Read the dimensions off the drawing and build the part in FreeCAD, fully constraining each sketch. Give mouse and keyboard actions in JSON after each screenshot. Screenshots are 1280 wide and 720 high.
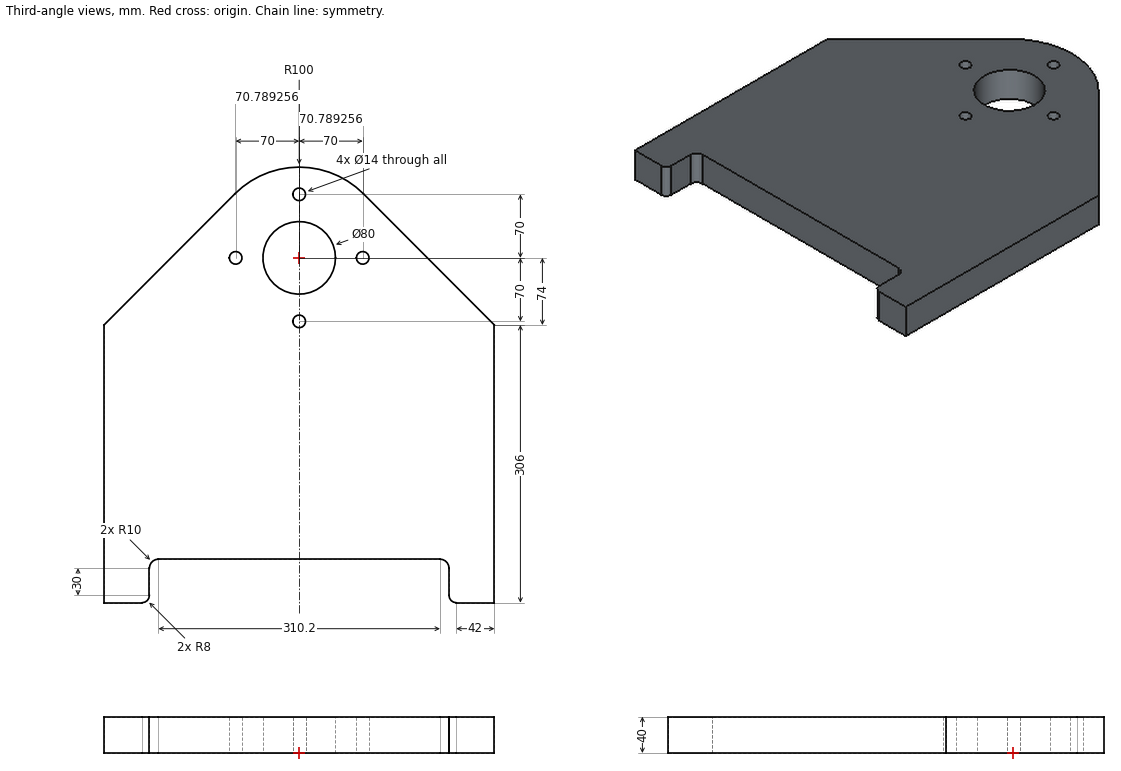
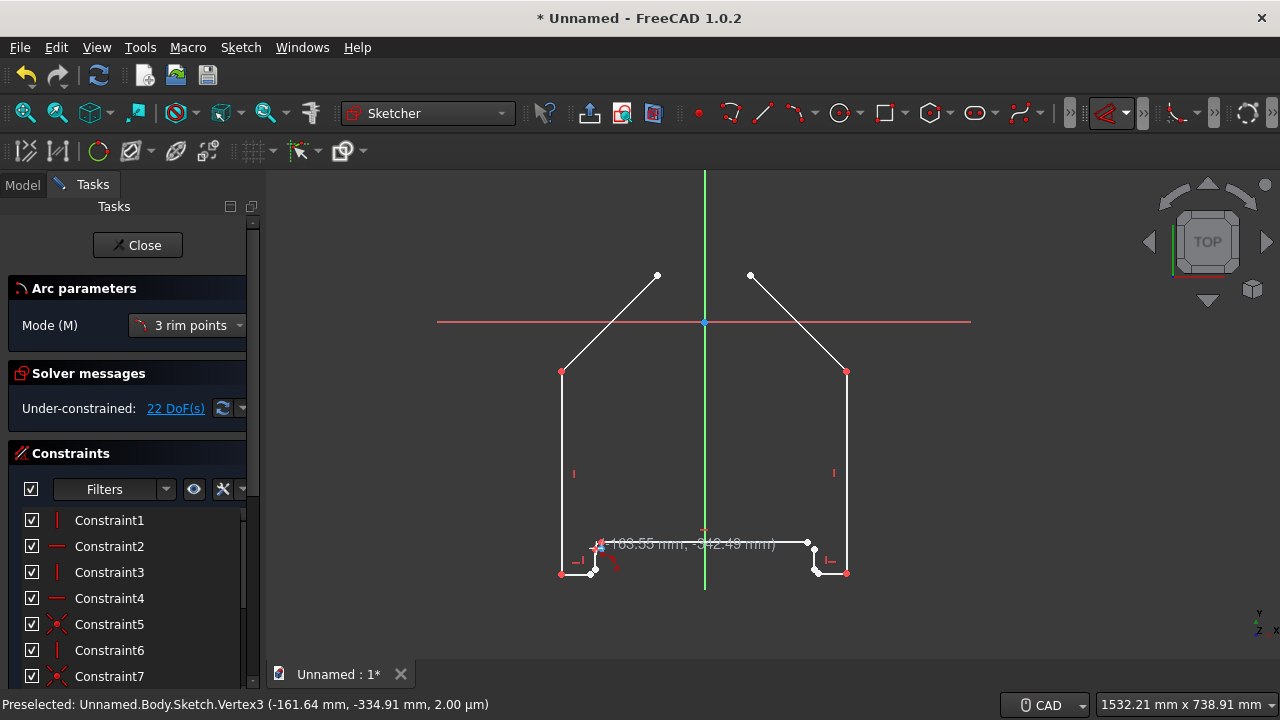
{"action": "scroll", "coordinate": [807, 542], "scroll_direction": "up", "scroll_amount": 3}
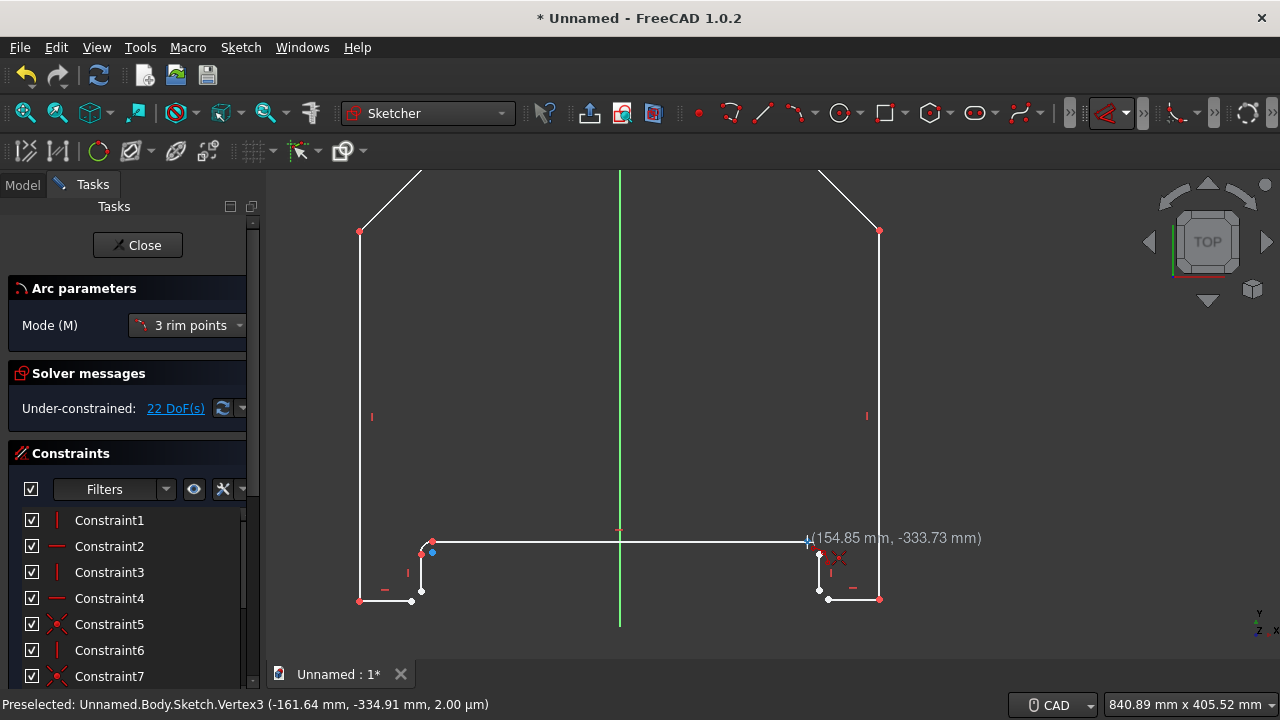
{"action": "left_click", "coordinate": [807, 542]}
{"action": "left_click", "coordinate": [819, 555]}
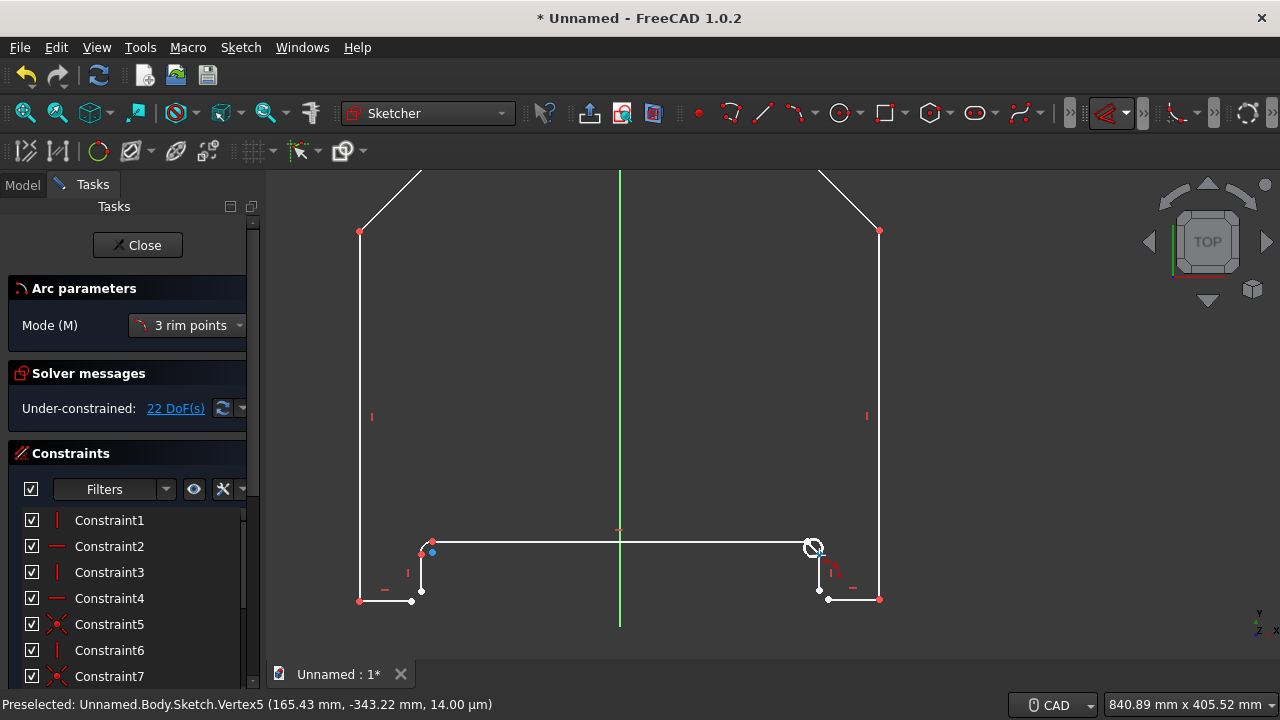
{"action": "scroll", "coordinate": [815, 545], "scroll_direction": "up", "scroll_amount": 8}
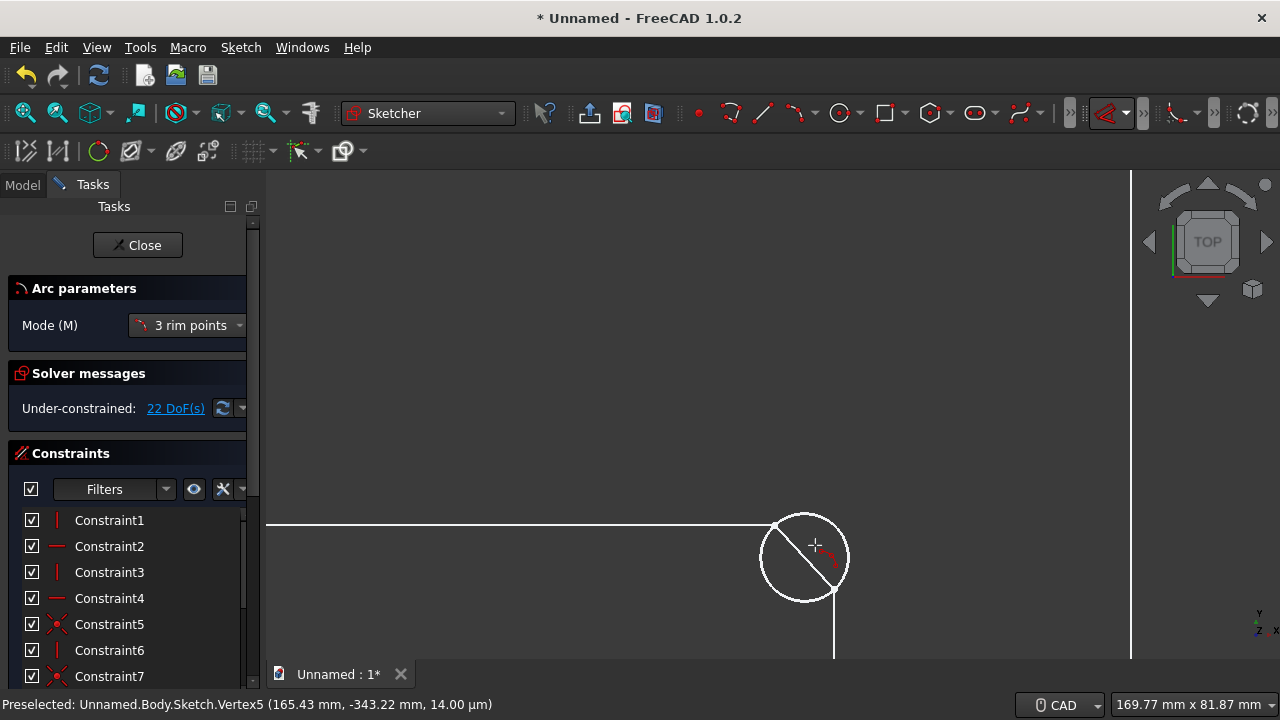
{"action": "left_click", "coordinate": [815, 540]}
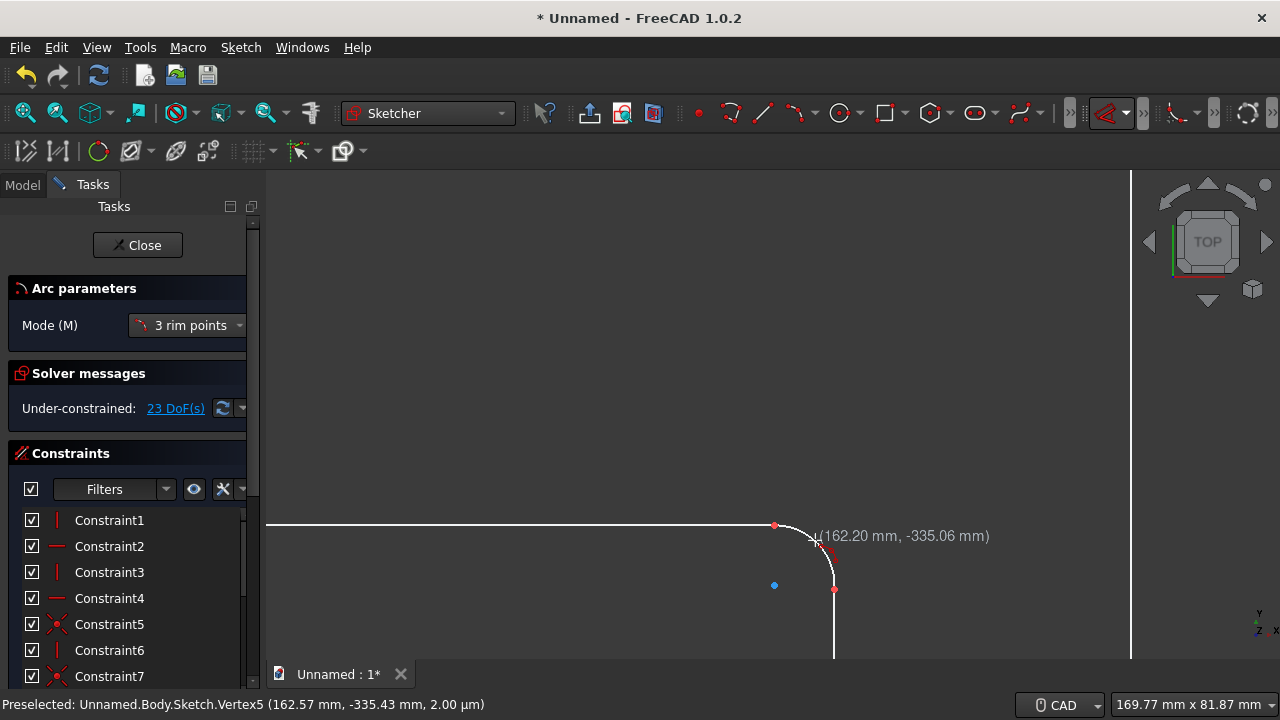
{"action": "scroll", "coordinate": [811, 544], "scroll_direction": "down", "scroll_amount": 11}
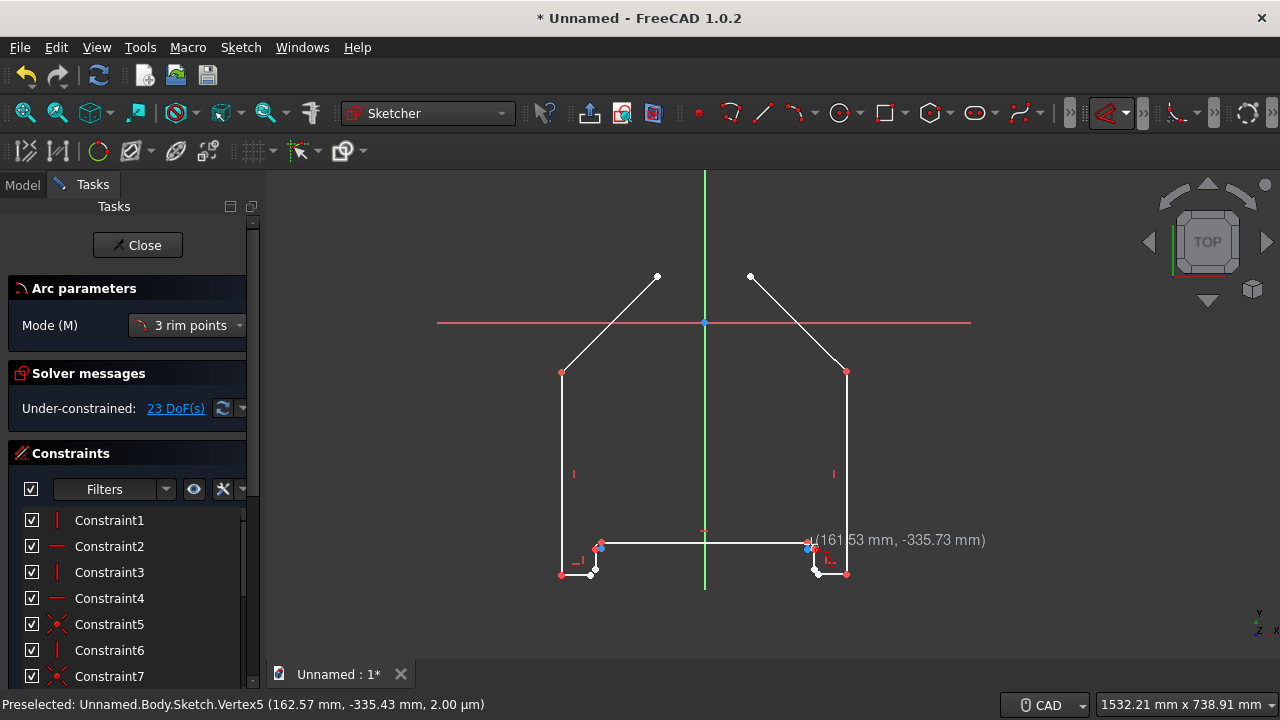
{"action": "scroll", "coordinate": [814, 569], "scroll_direction": "up", "scroll_amount": 4}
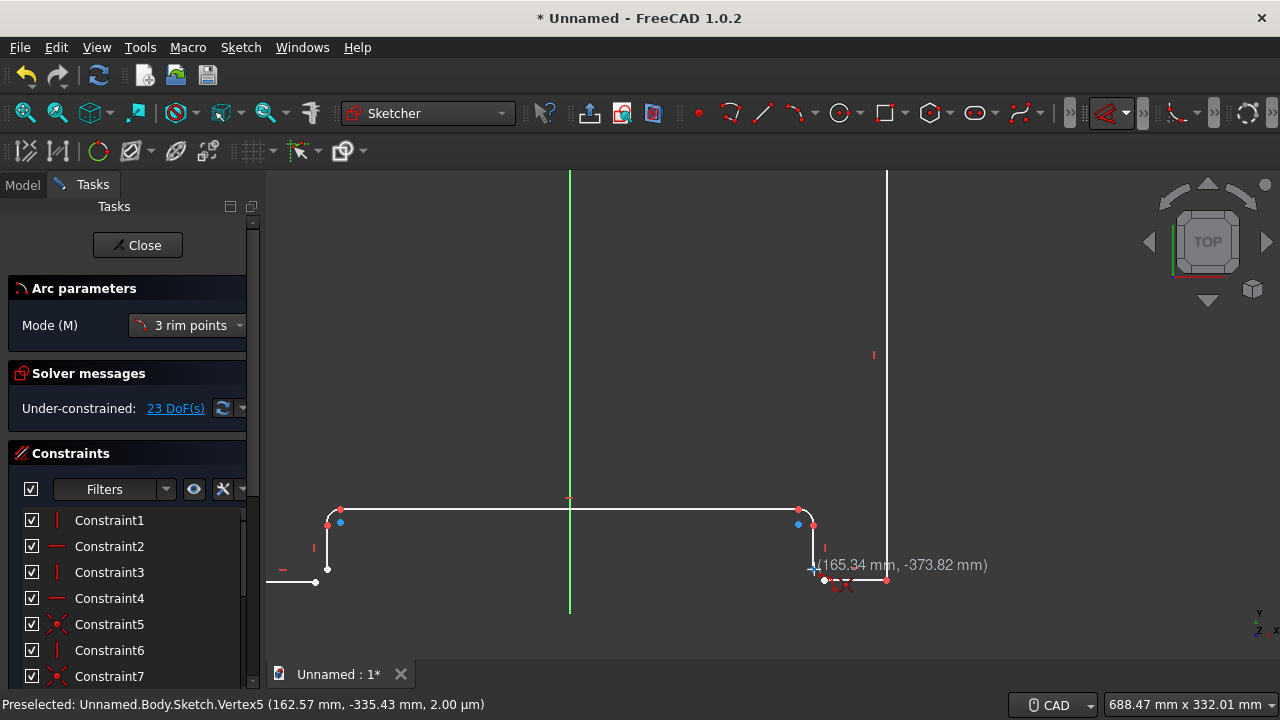
{"action": "left_click", "coordinate": [813, 569]}
{"action": "left_click", "coordinate": [824, 580]}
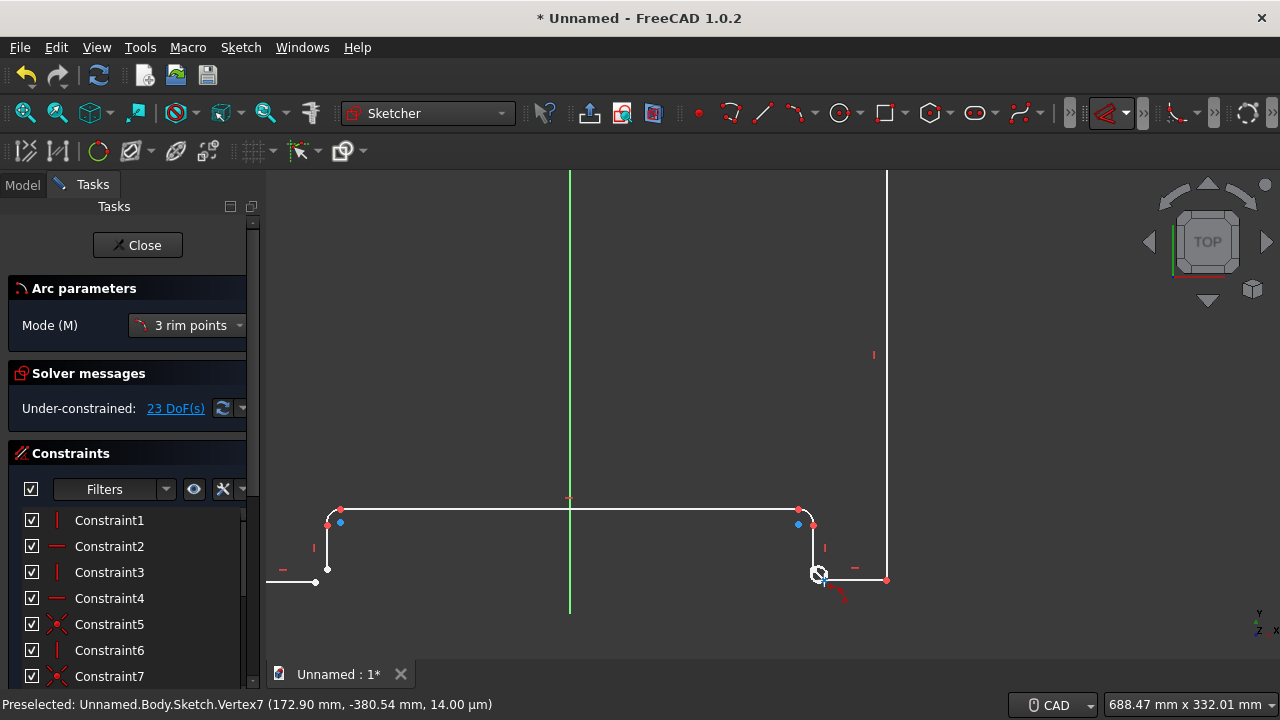
{"action": "scroll", "coordinate": [816, 576], "scroll_direction": "up", "scroll_amount": 8}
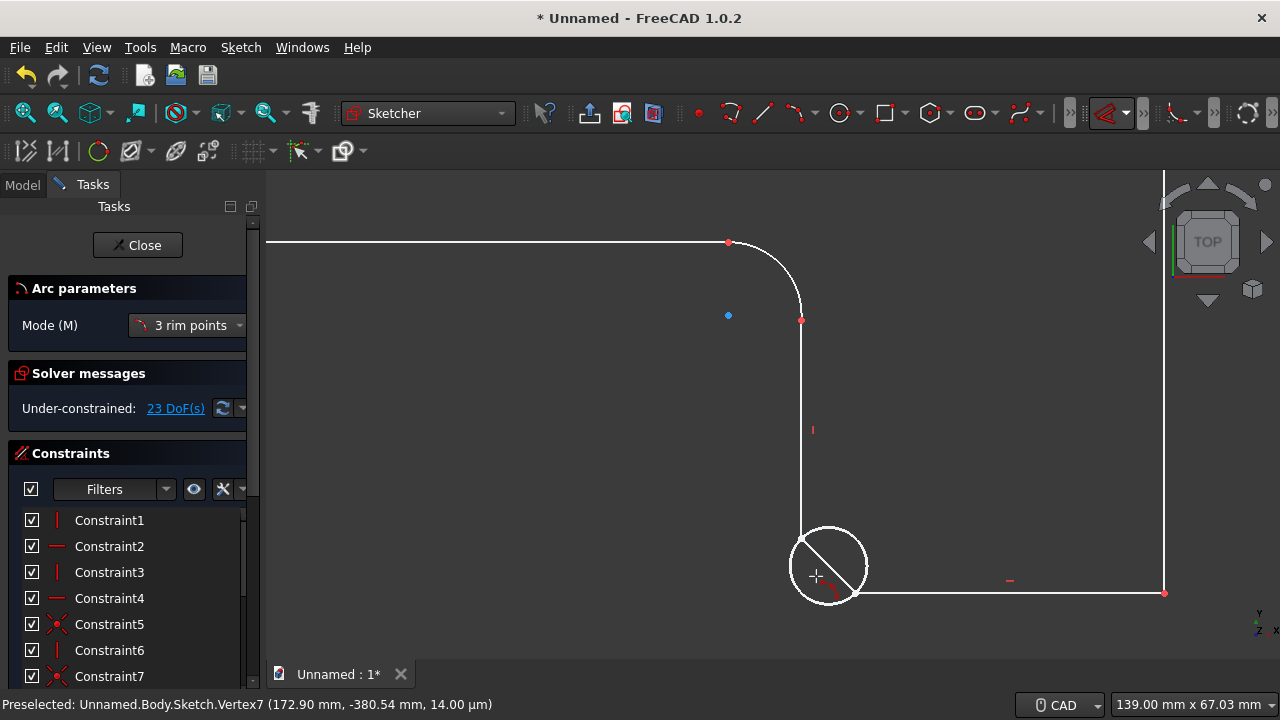
{"action": "left_click", "coordinate": [816, 572]}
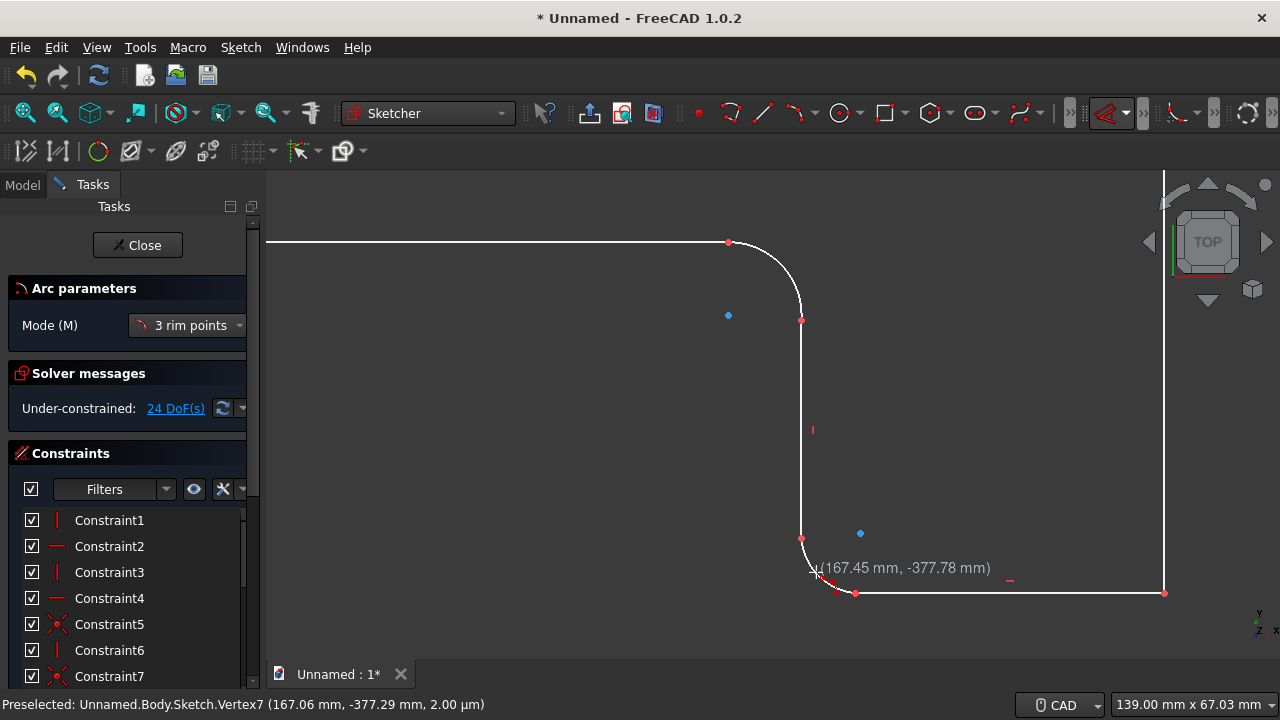
{"action": "scroll", "coordinate": [815, 572], "scroll_direction": "down", "scroll_amount": 12}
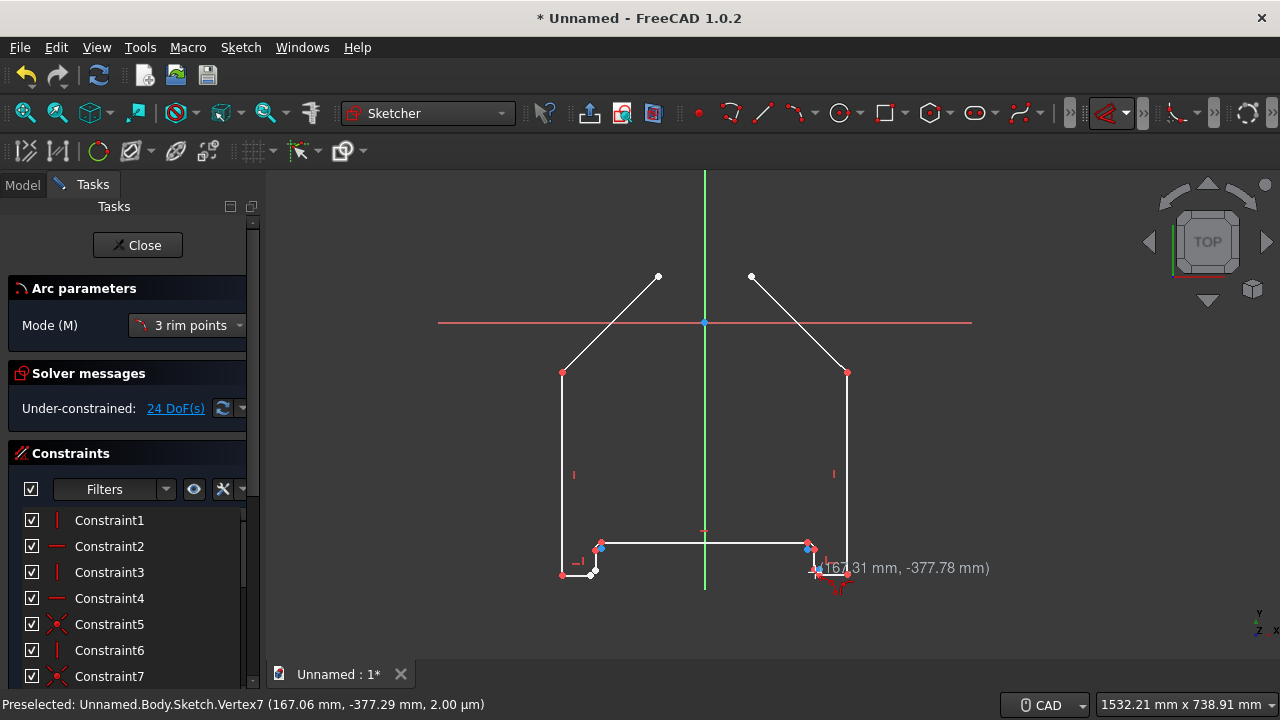
{"action": "left_click", "coordinate": [751, 277]}
{"action": "left_click", "coordinate": [658, 277]}
{"action": "left_click", "coordinate": [725, 260]}